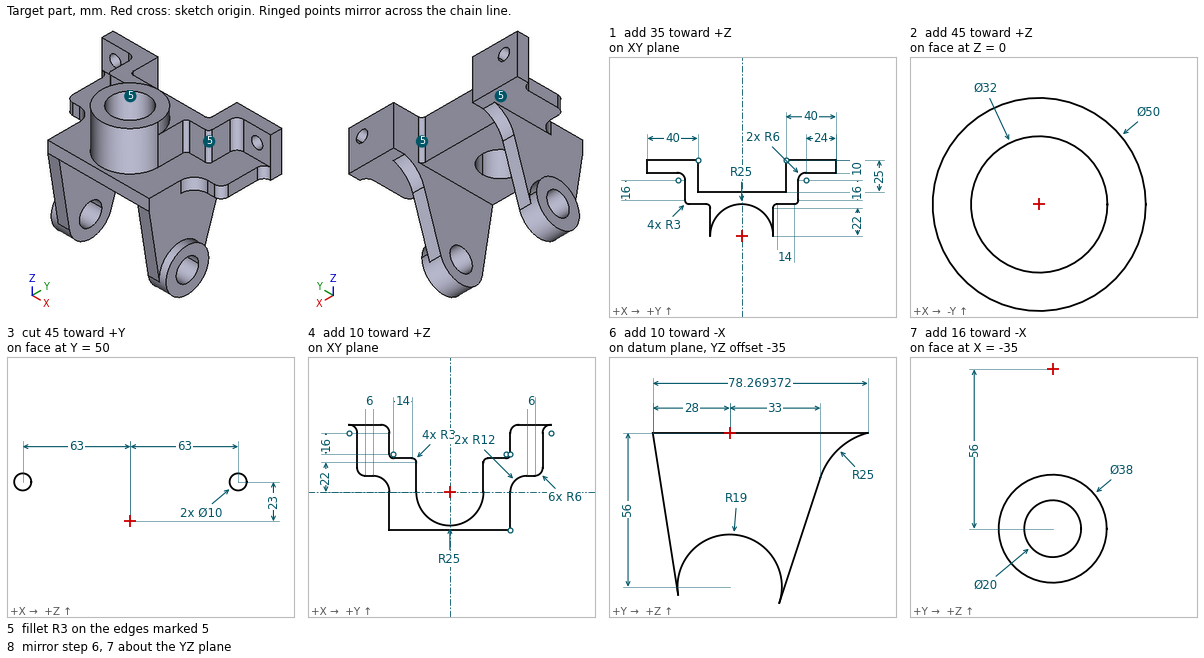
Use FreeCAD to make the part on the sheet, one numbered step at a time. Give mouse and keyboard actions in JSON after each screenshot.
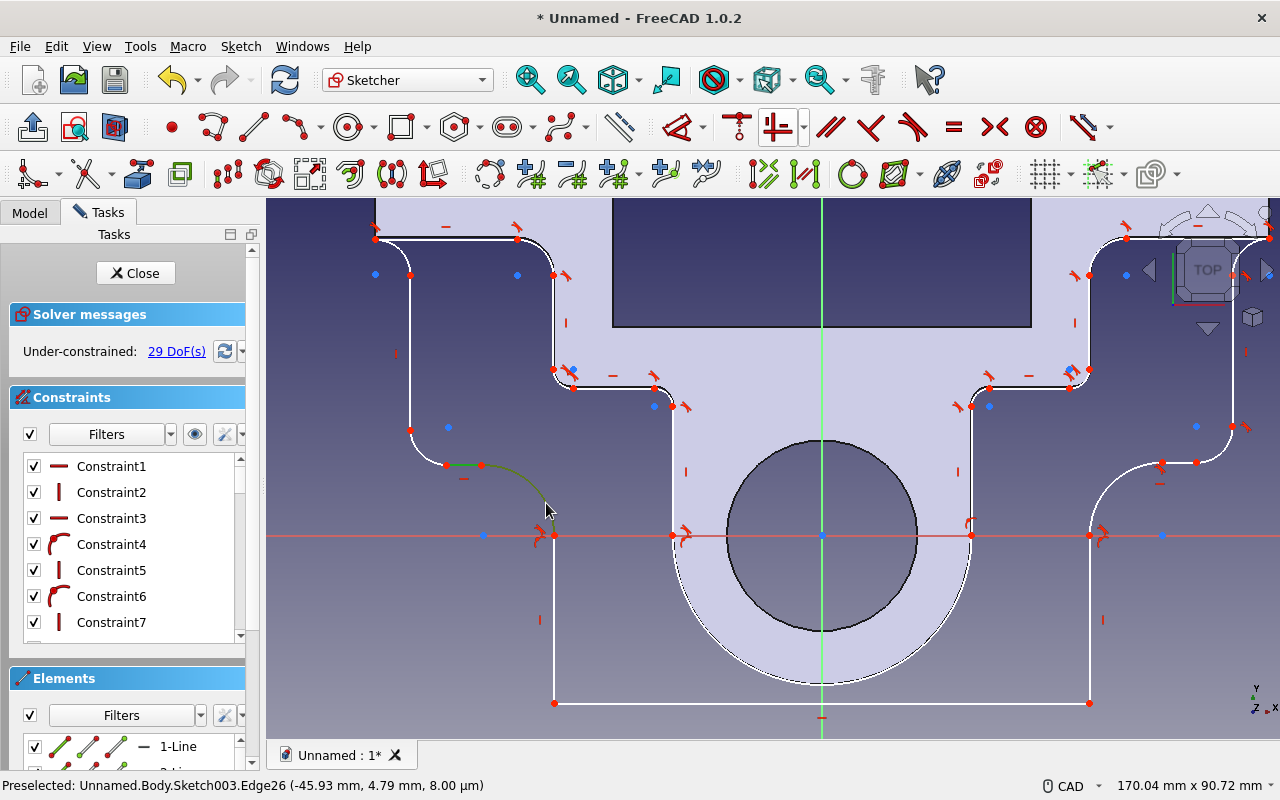
{"action": "left_click", "coordinate": [913, 128]}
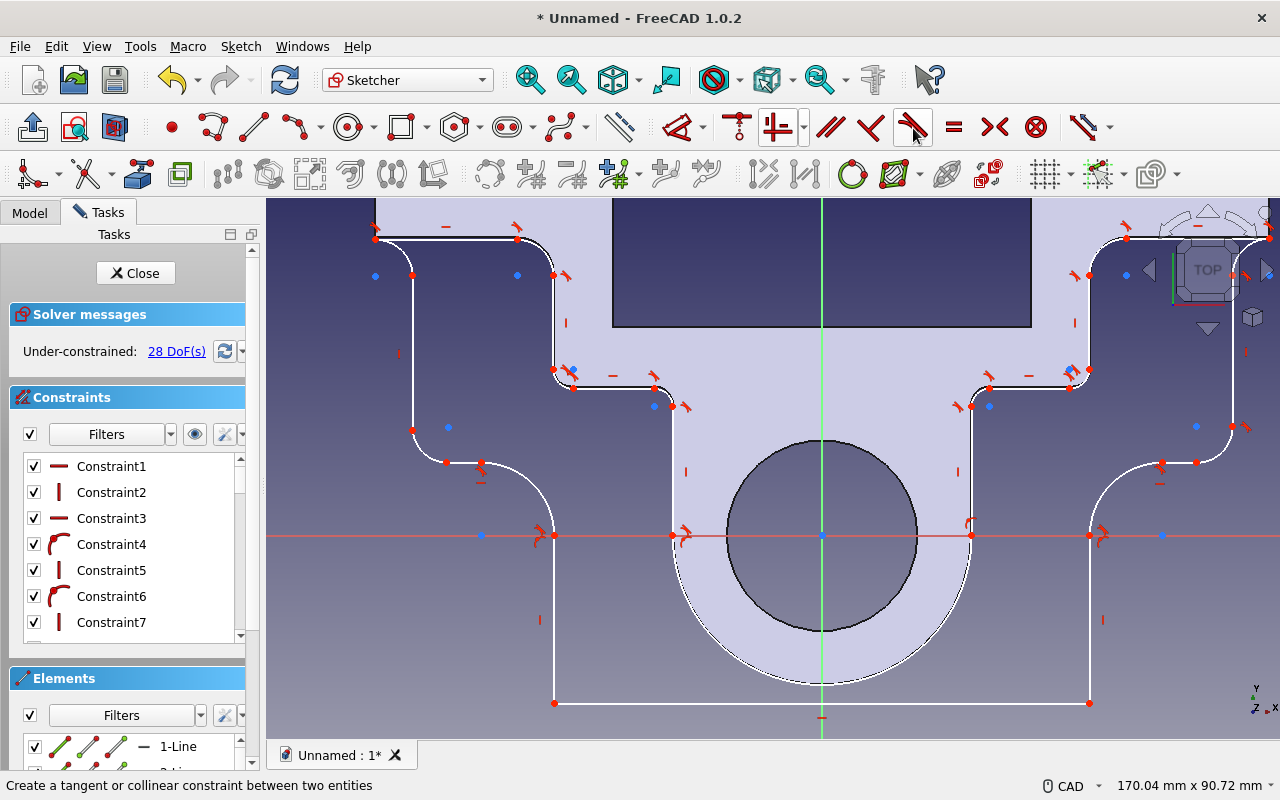
{"action": "scroll", "coordinate": [471, 463], "scroll_direction": "up", "scroll_amount": 2}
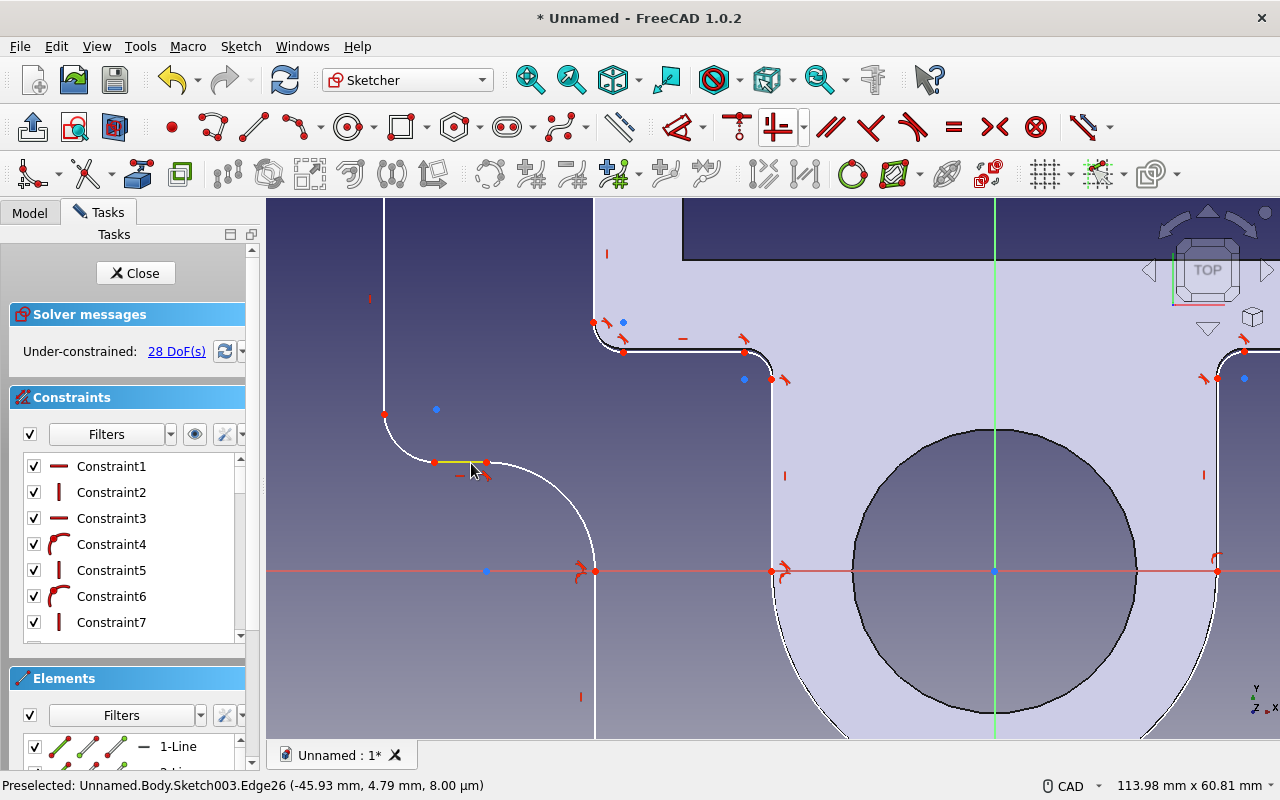
{"action": "left_click", "coordinate": [471, 462]}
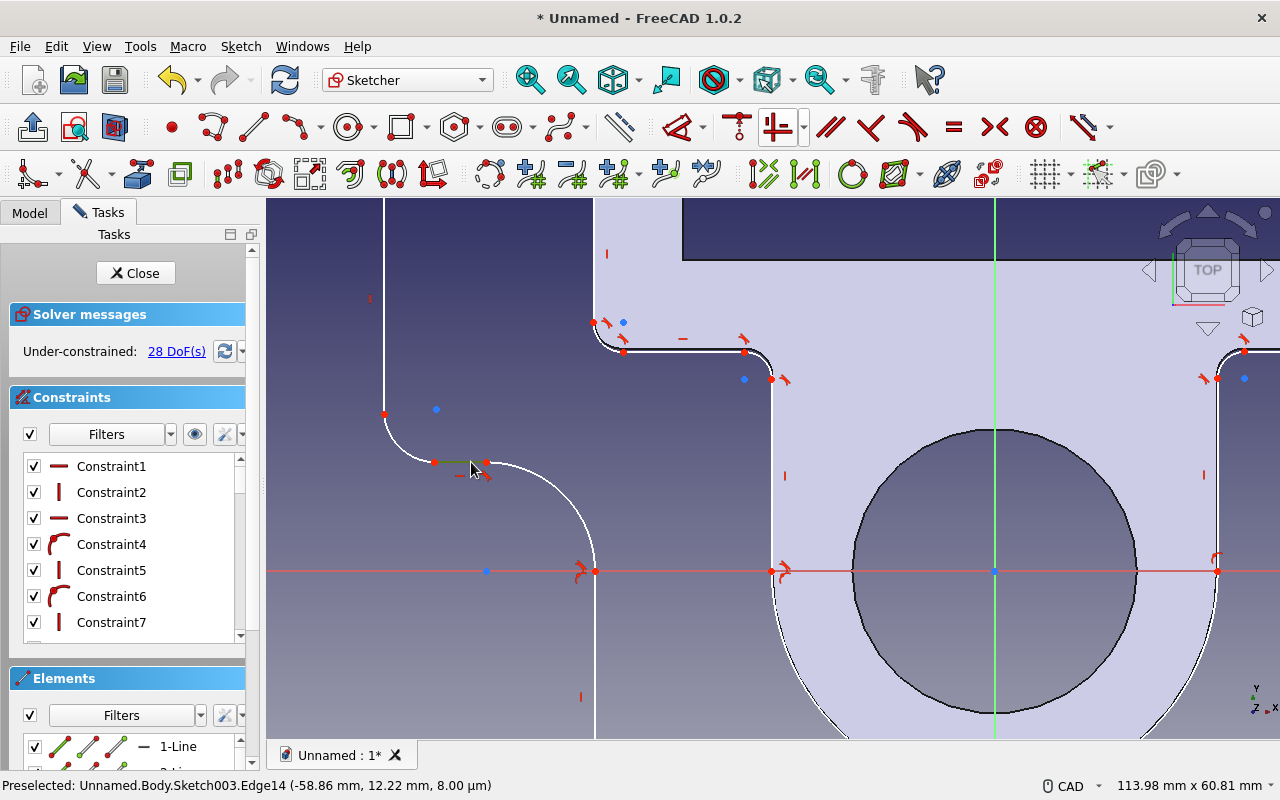
{"action": "left_click", "coordinate": [391, 436]}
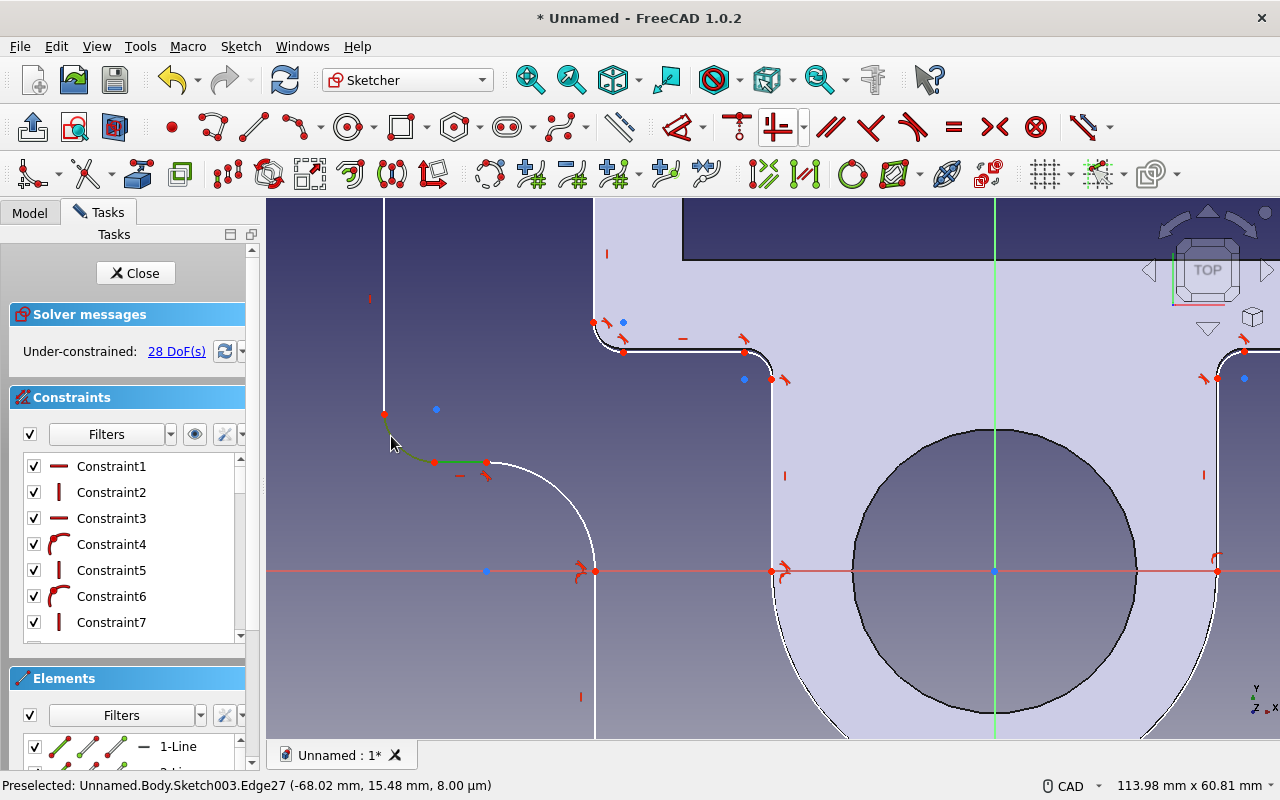
{"action": "left_click", "coordinate": [913, 128]}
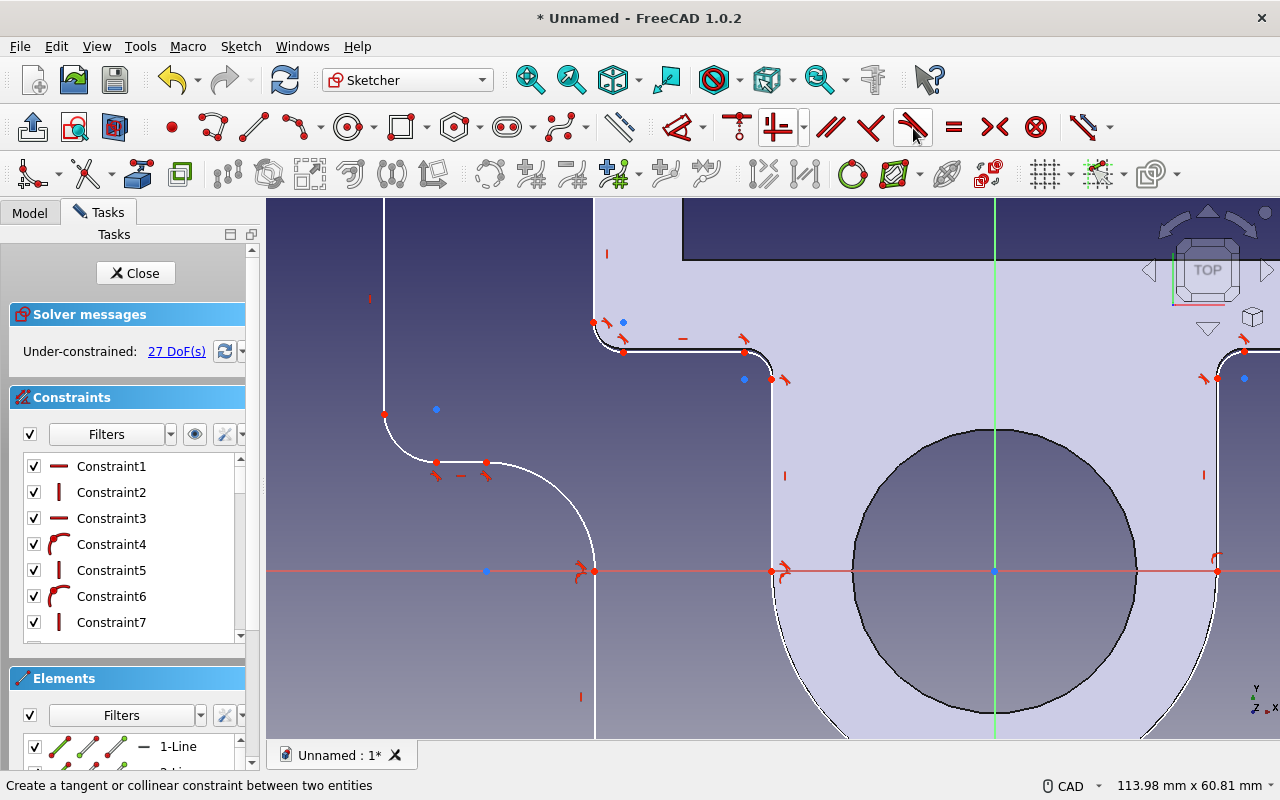
{"action": "left_click", "coordinate": [384, 345]}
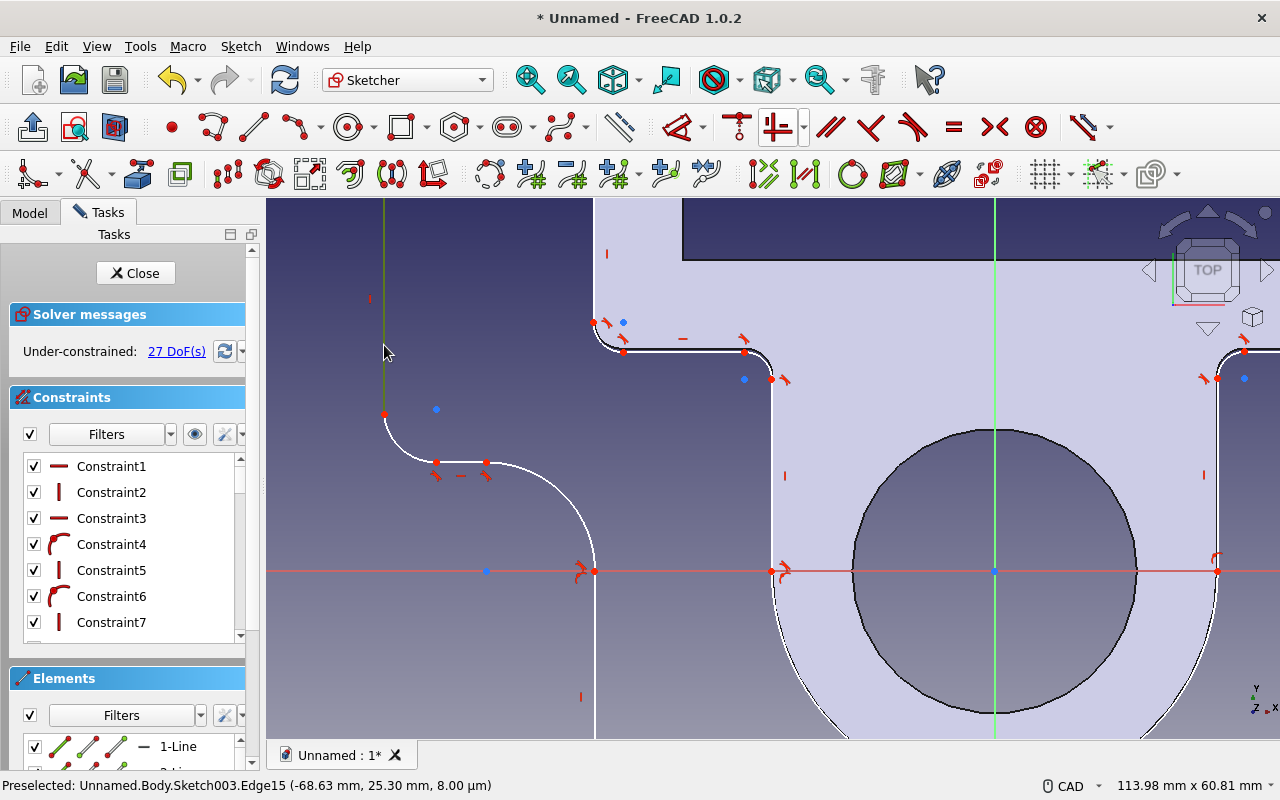
{"action": "left_click", "coordinate": [391, 437]}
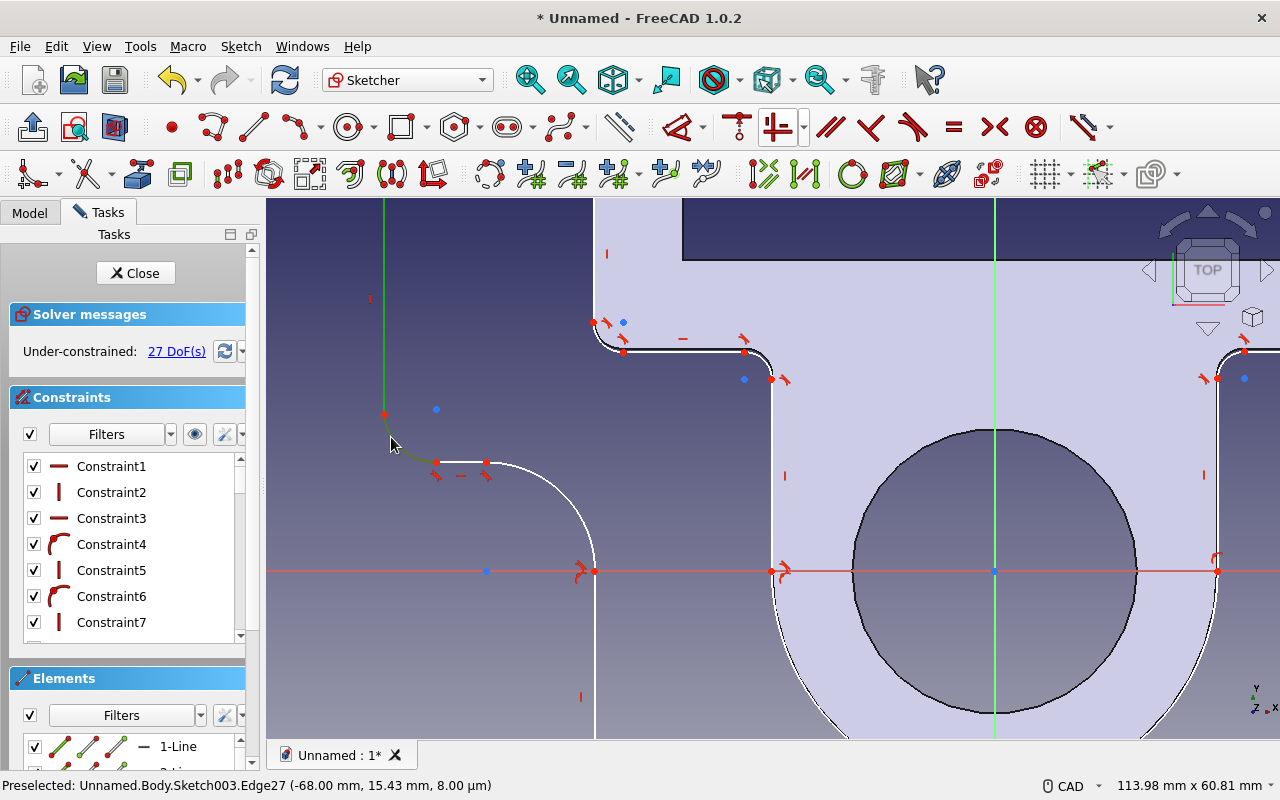
{"action": "left_click", "coordinate": [913, 128]}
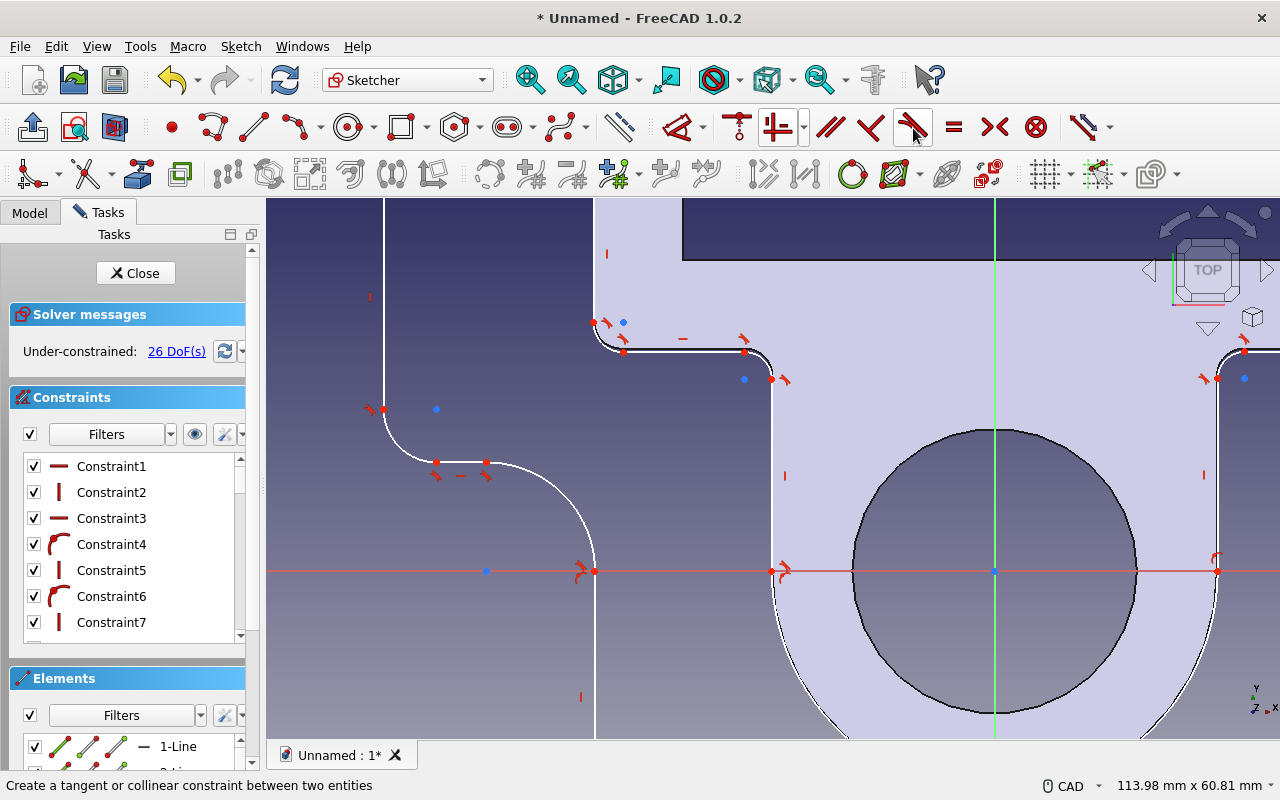
{"action": "left_click", "coordinate": [384, 342]}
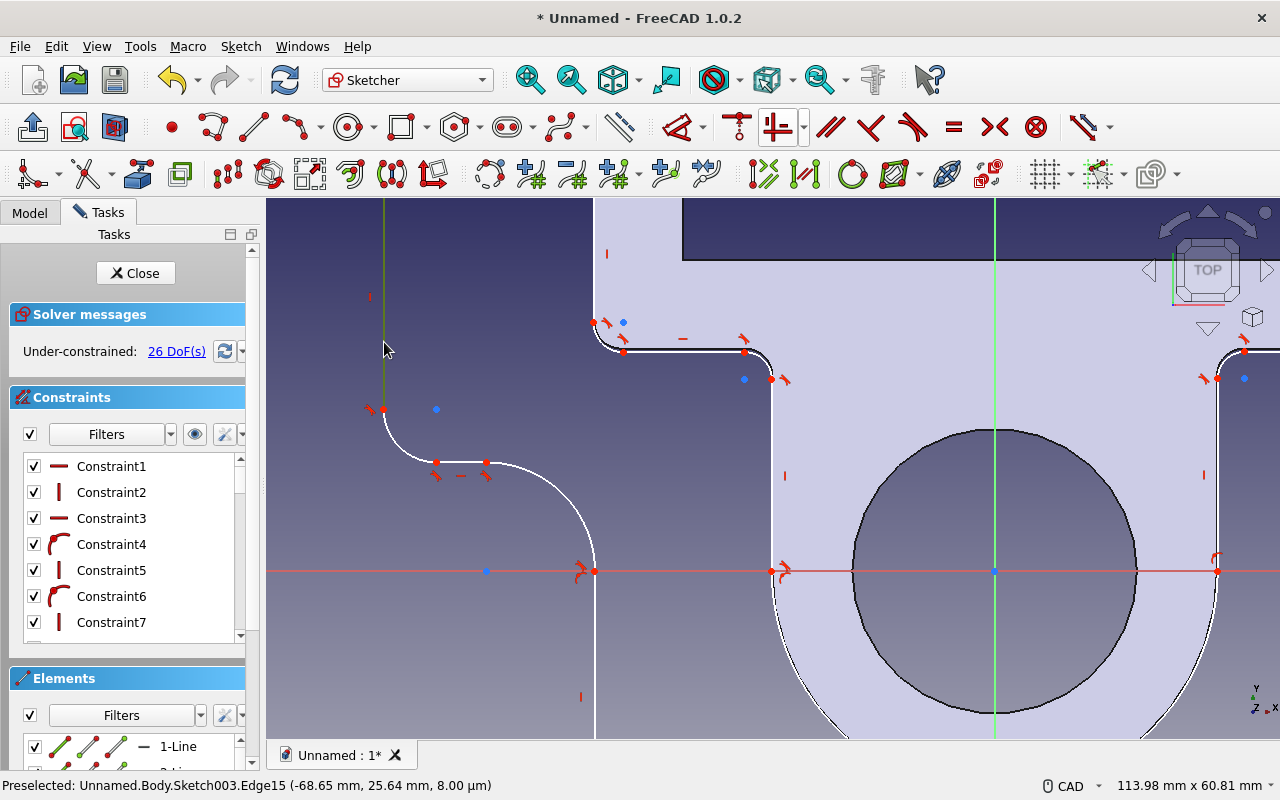
{"action": "scroll", "coordinate": [468, 465], "scroll_direction": "down", "scroll_amount": 4}